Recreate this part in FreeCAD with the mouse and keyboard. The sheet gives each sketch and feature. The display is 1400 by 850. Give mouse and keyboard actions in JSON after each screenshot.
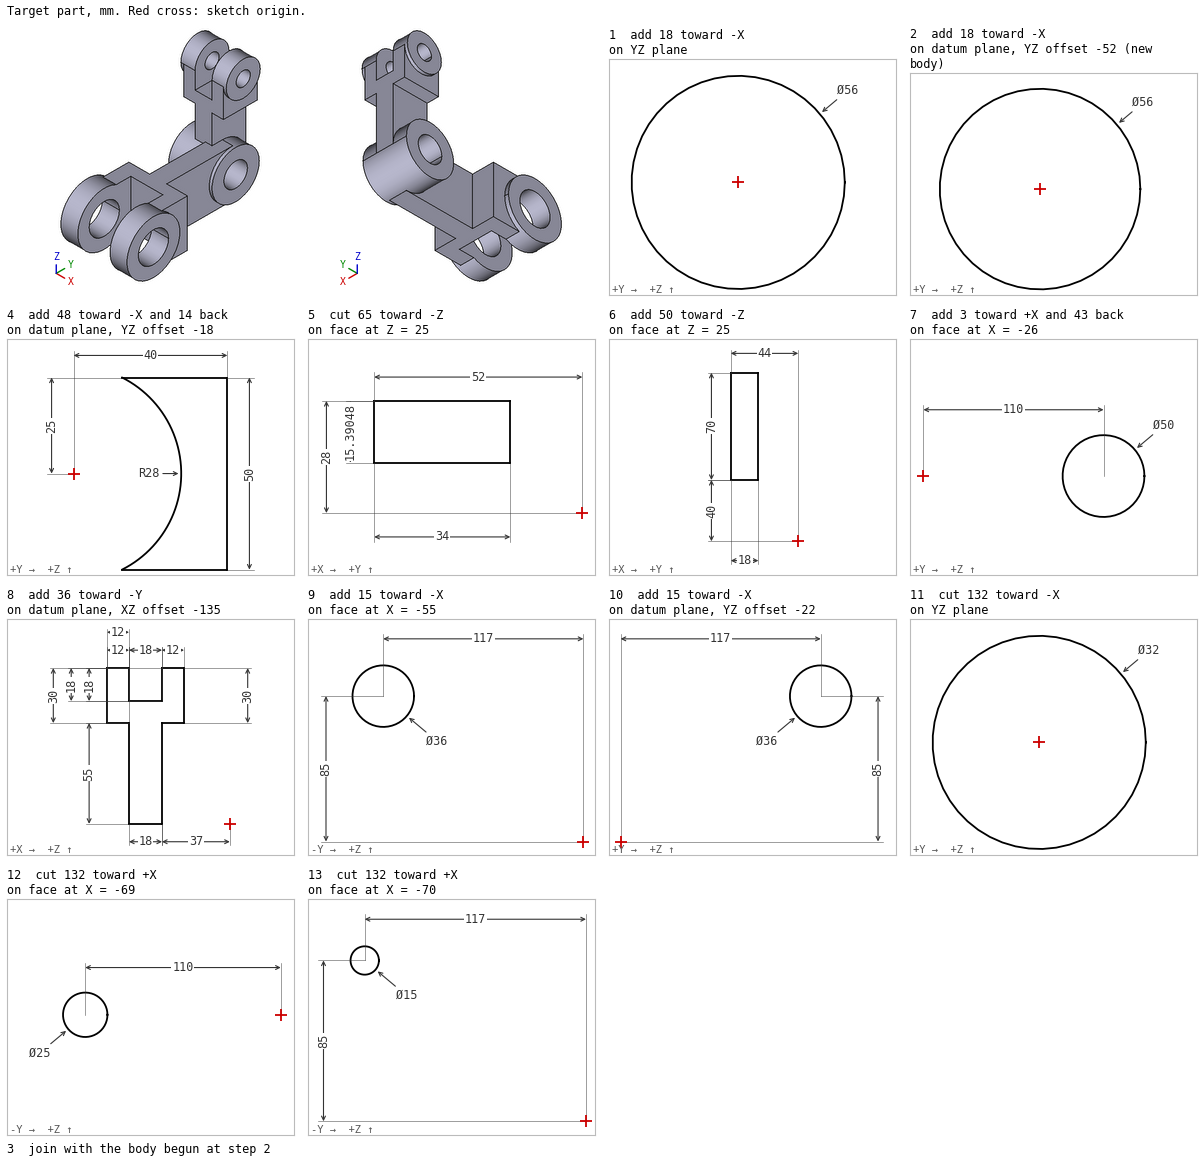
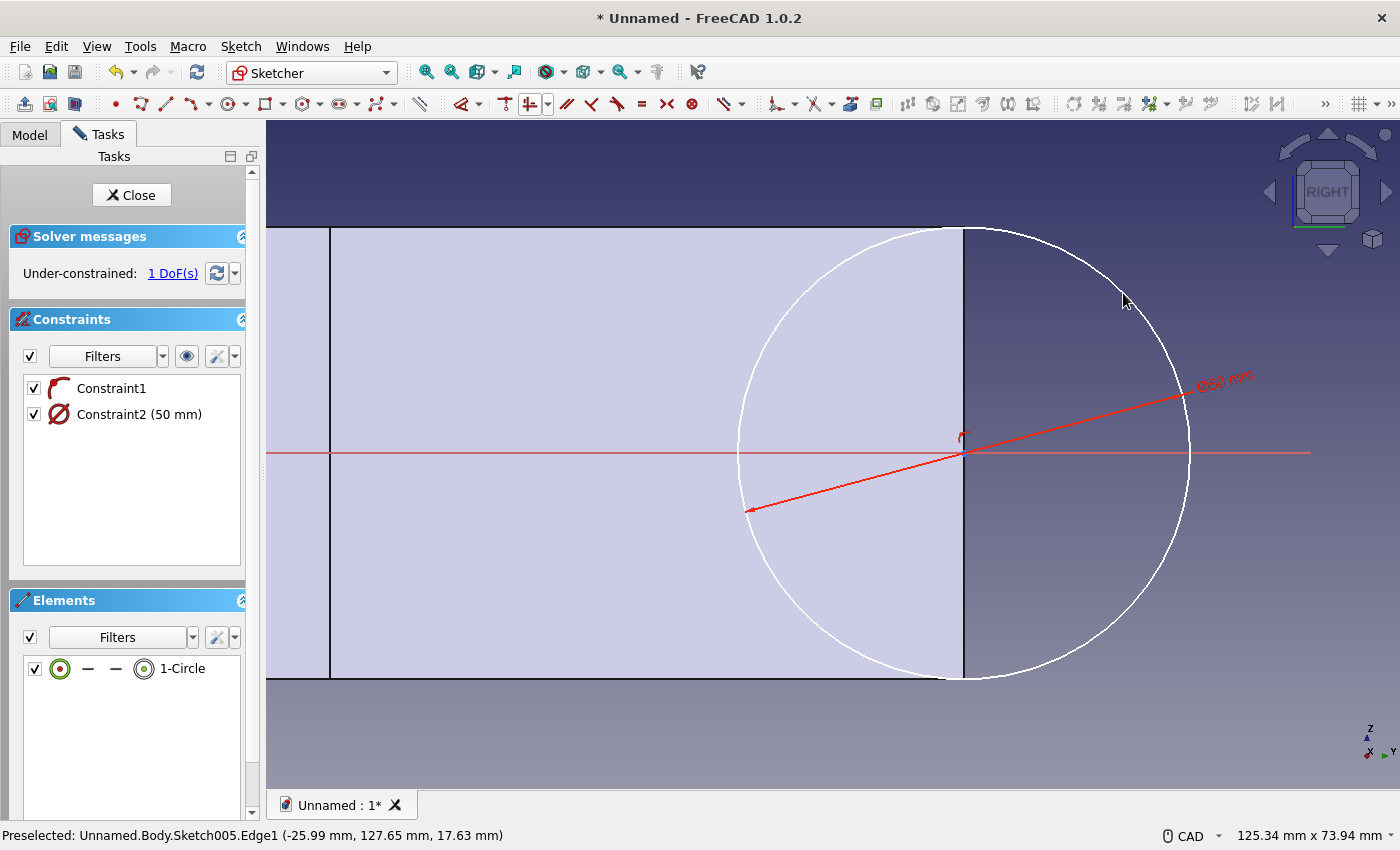
{"action": "left_click", "coordinate": [964, 453]}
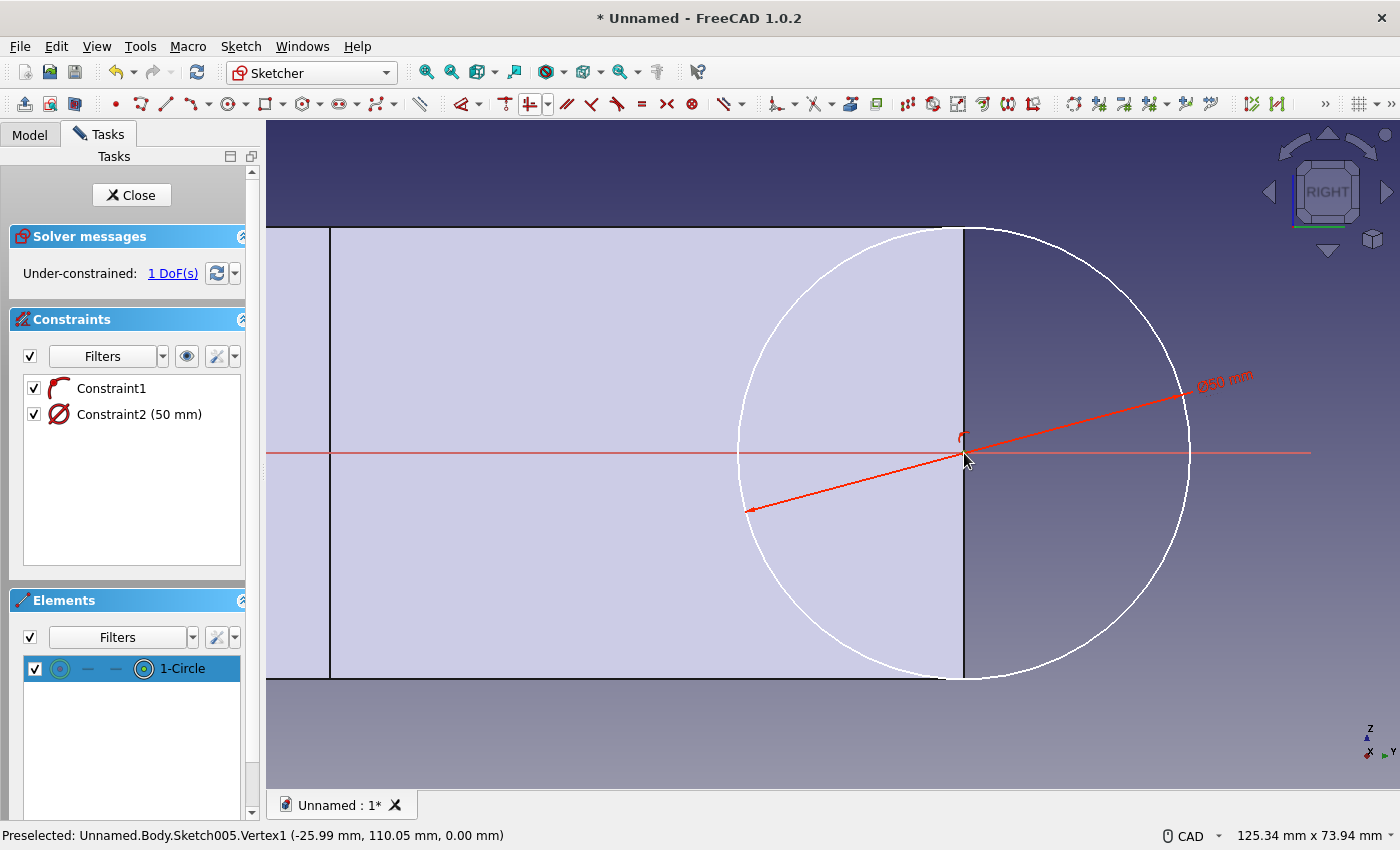
{"action": "key", "text": "l"}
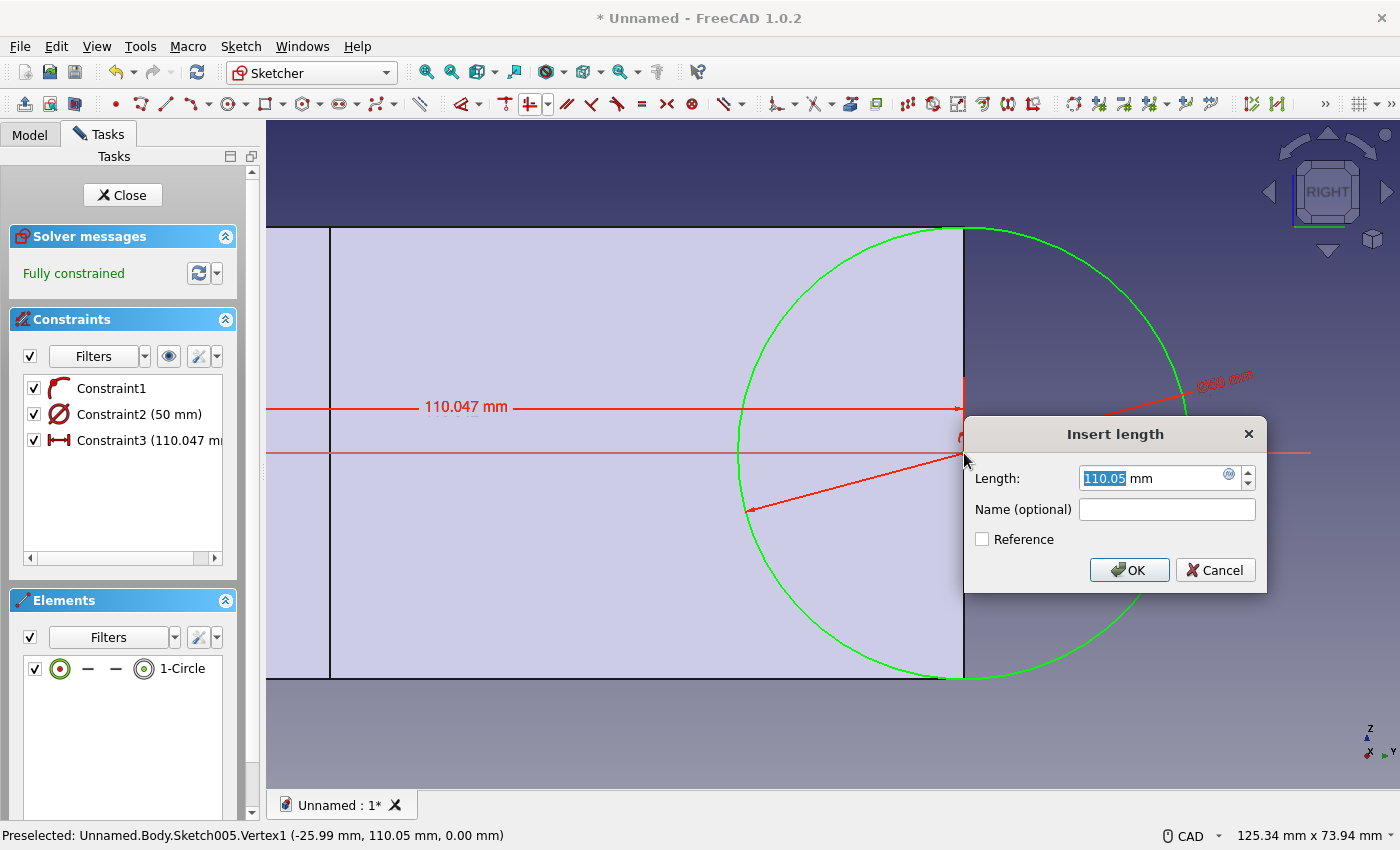
{"action": "type", "text": "110"}
{"action": "key", "text": "Return"}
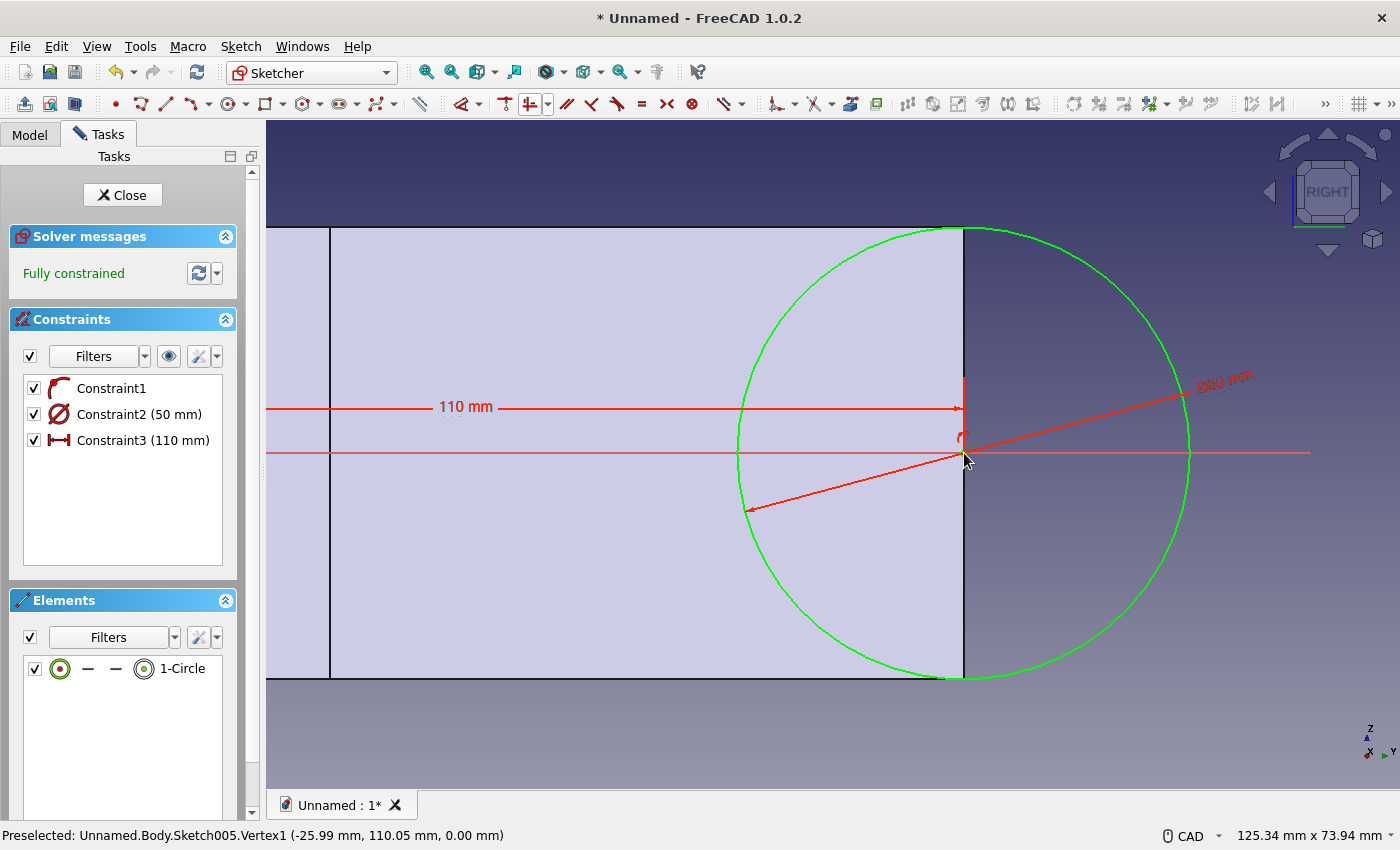
{"action": "left_click", "coordinate": [123, 195]}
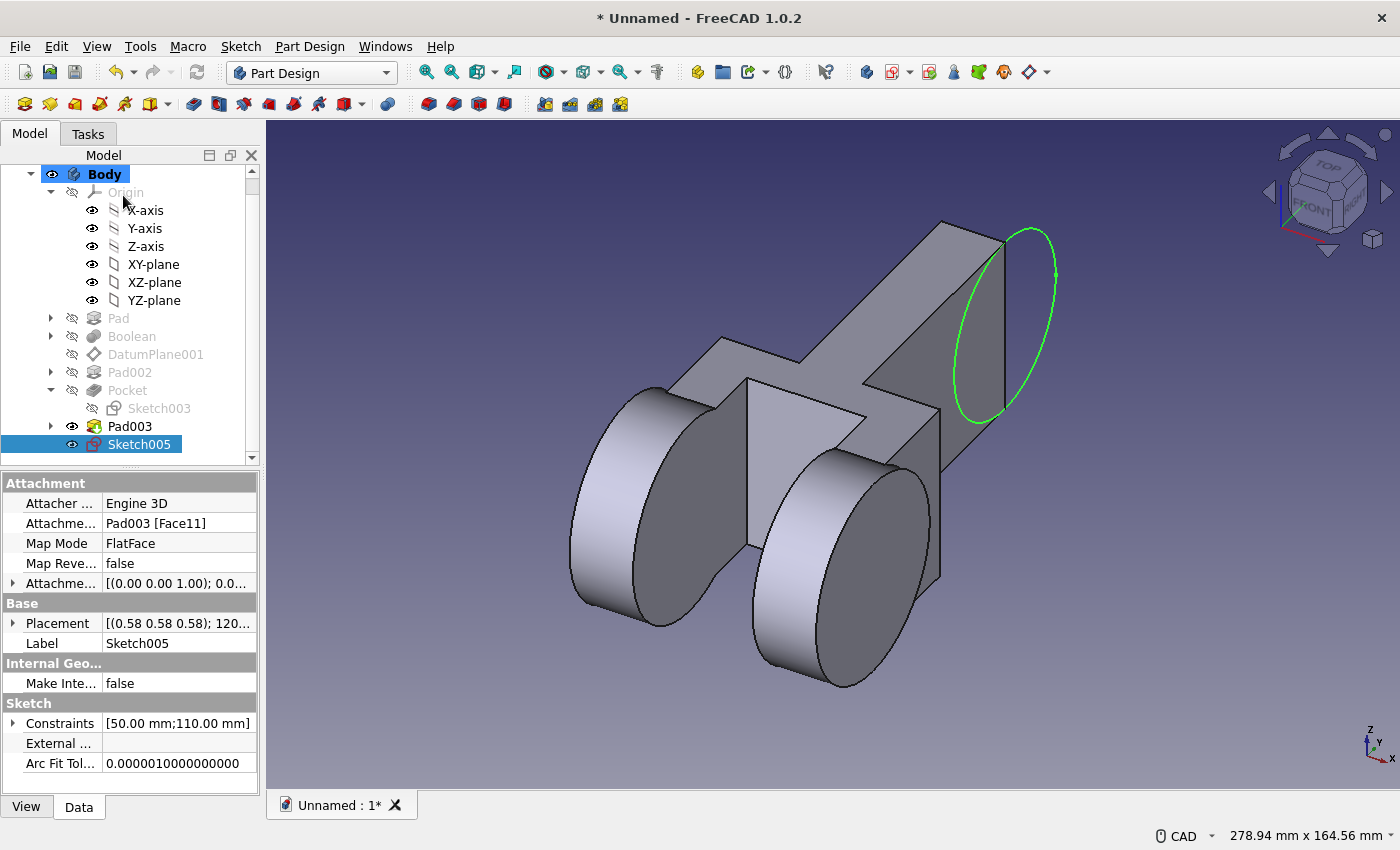
{"action": "left_click", "coordinate": [25, 104]}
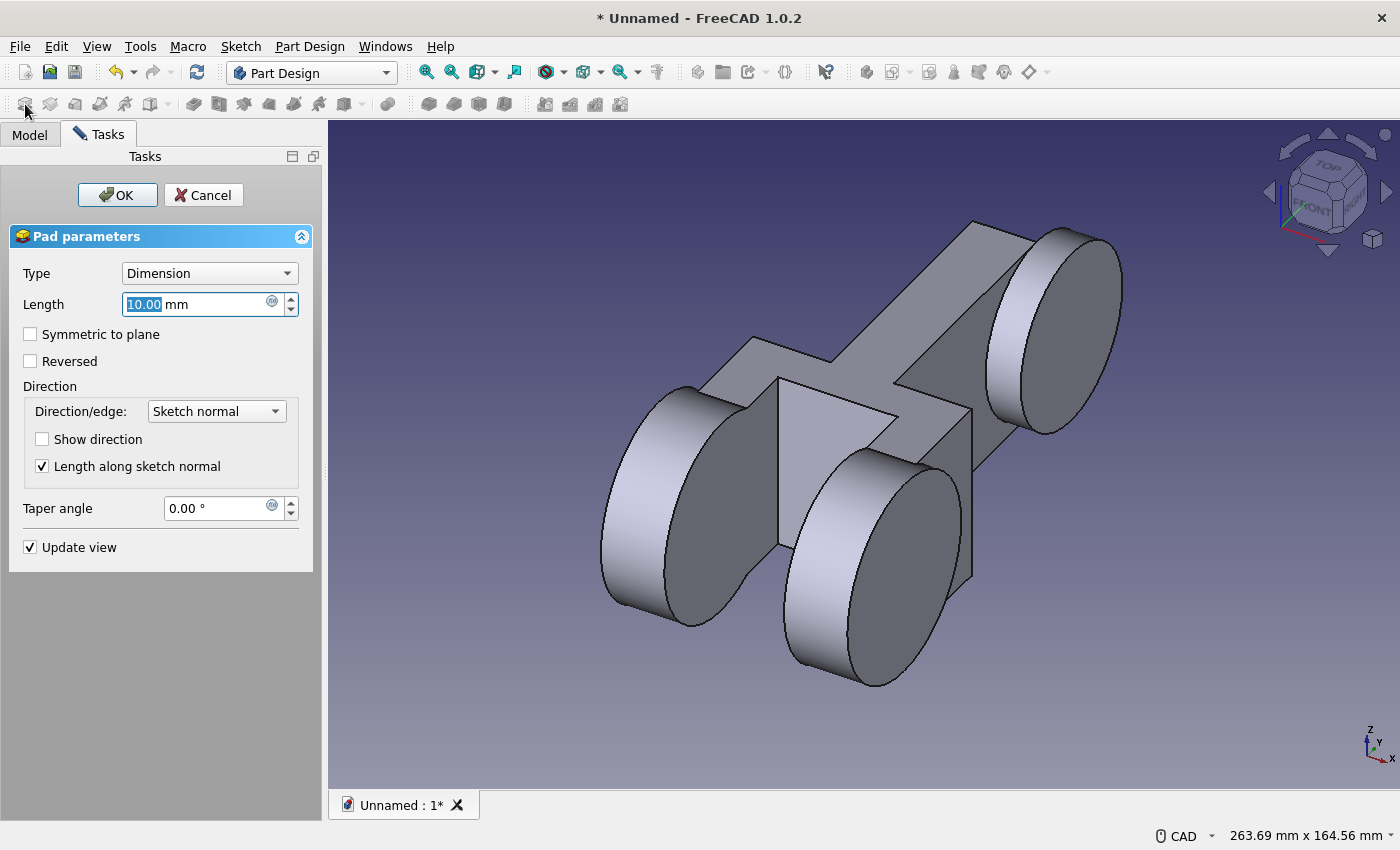
{"action": "left_click", "coordinate": [210, 274]}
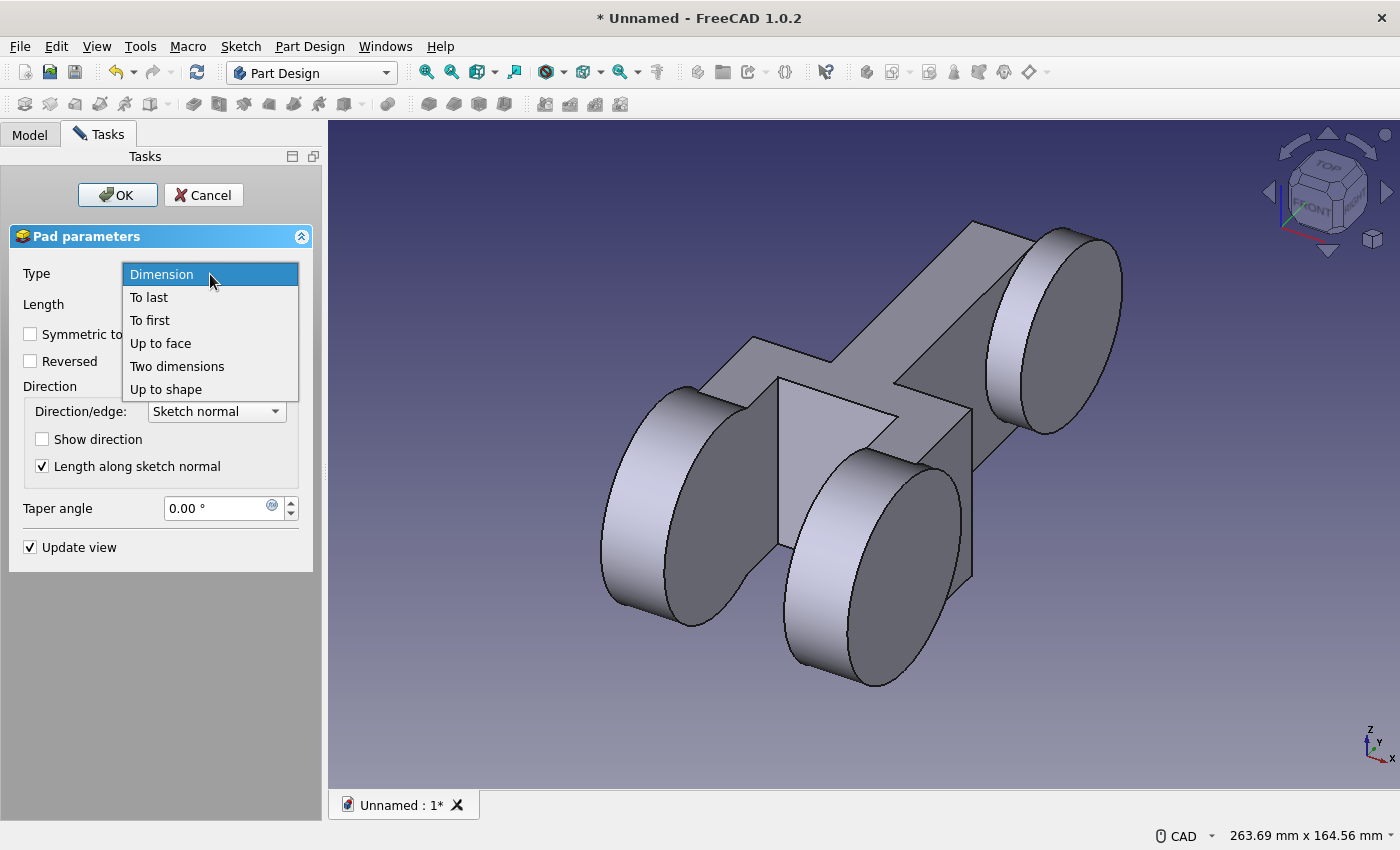
{"action": "left_click", "coordinate": [208, 366]}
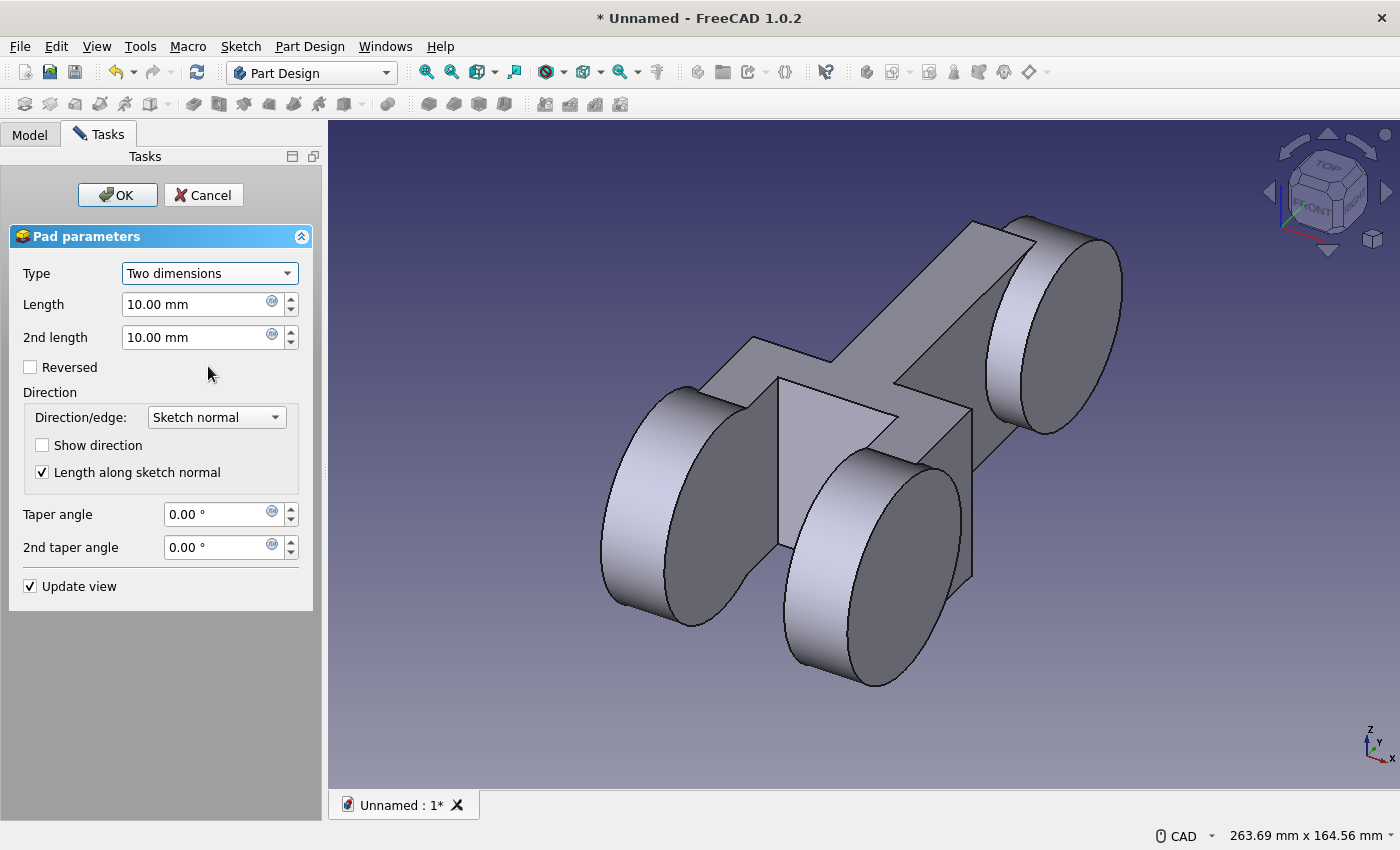
{"action": "triple_click", "coordinate": [204, 304]}